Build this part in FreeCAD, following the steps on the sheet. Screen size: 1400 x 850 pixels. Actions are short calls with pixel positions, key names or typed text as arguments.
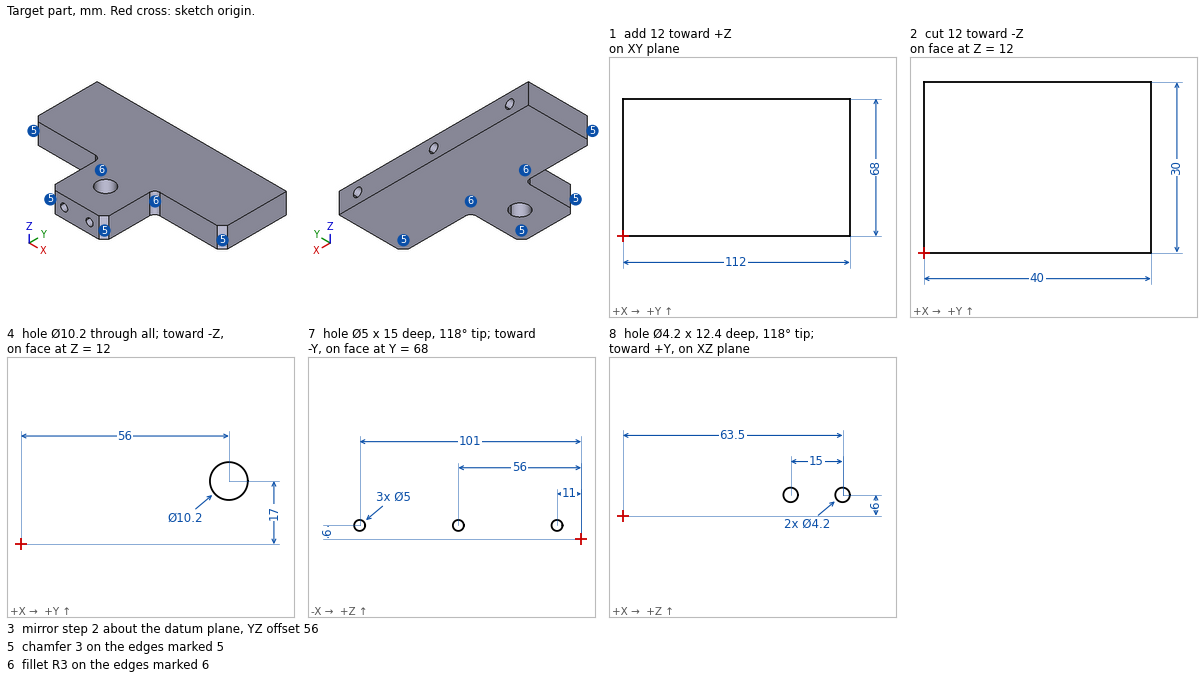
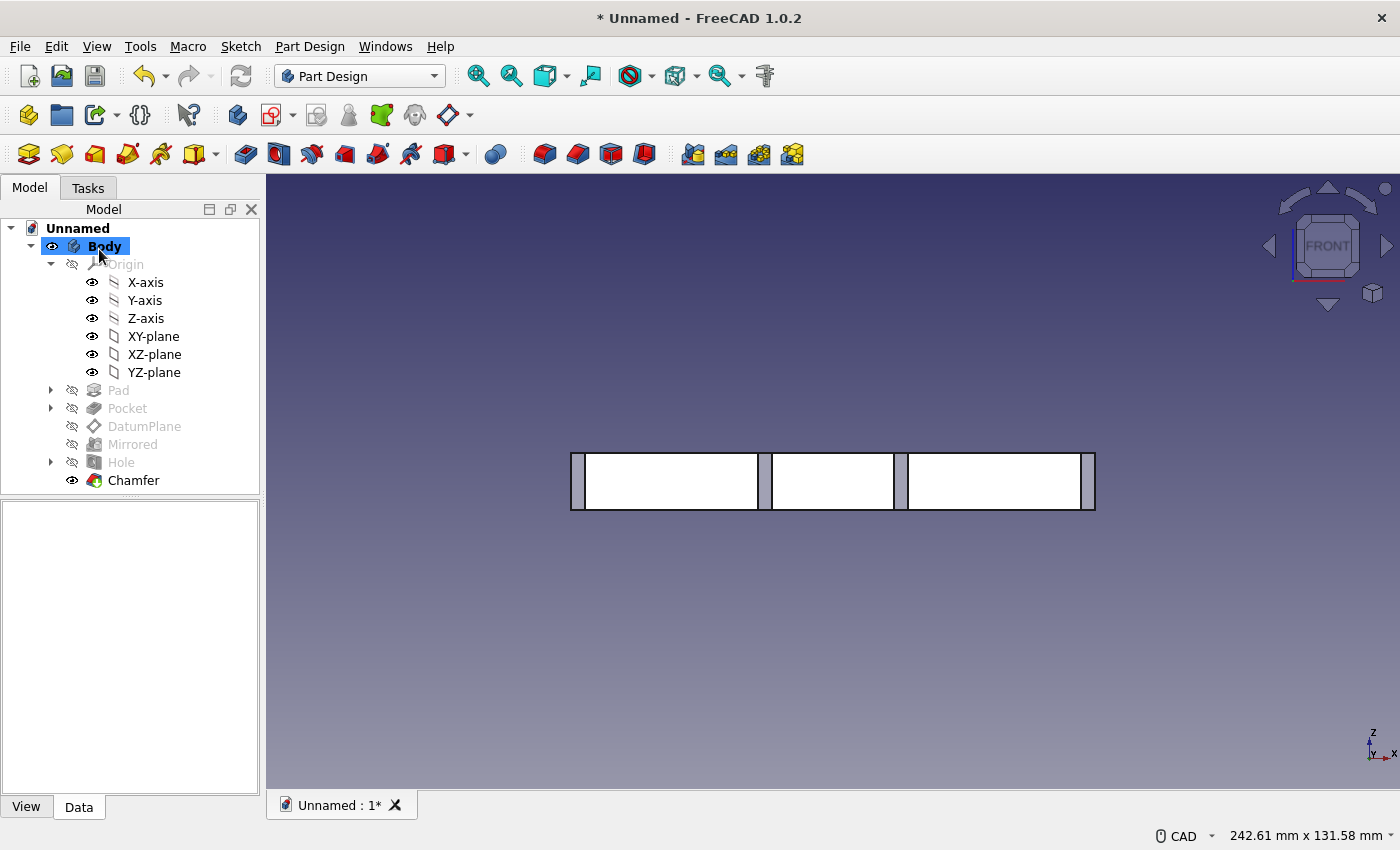
key(3)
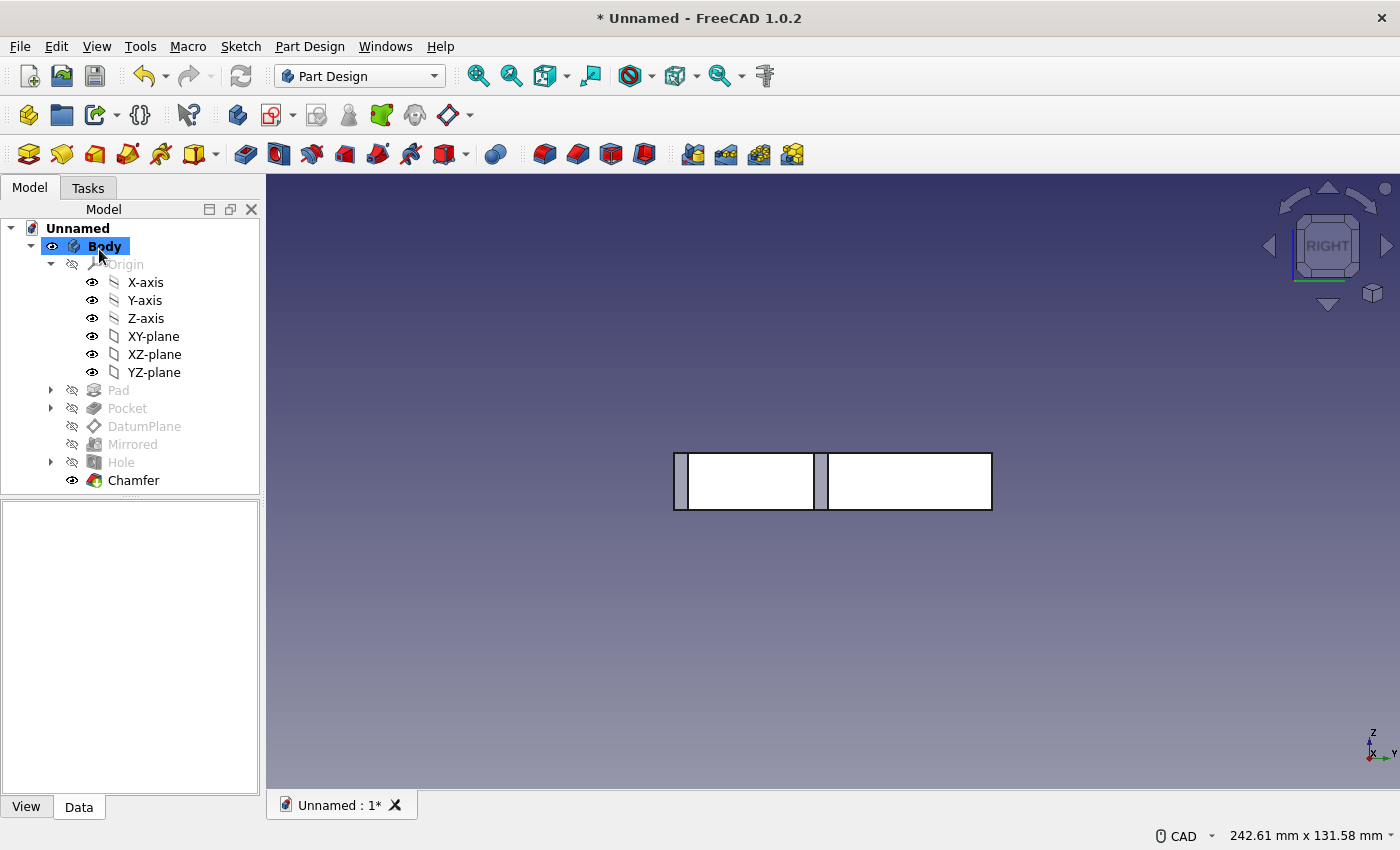
click(479, 76)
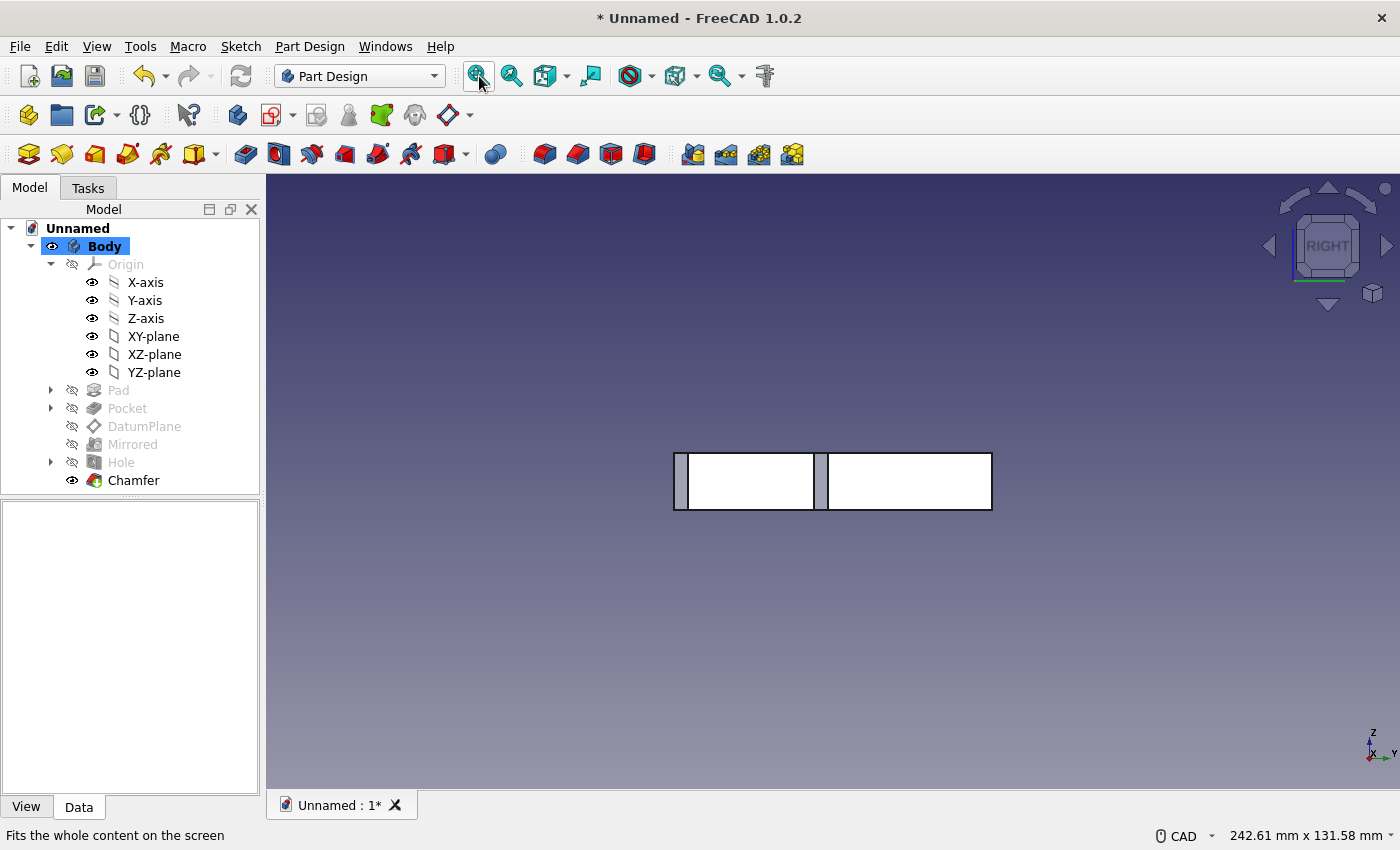
key(5)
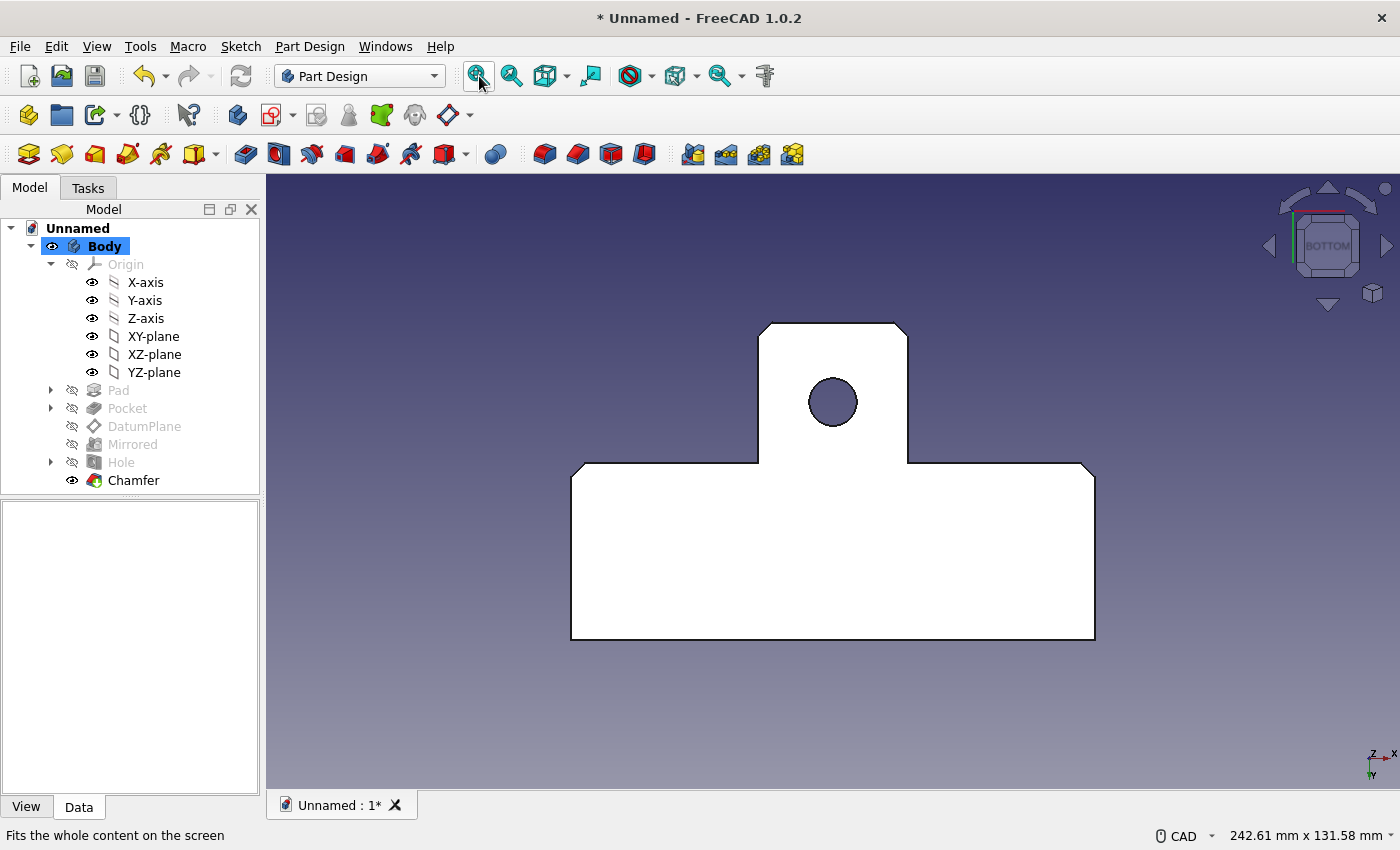
key(4)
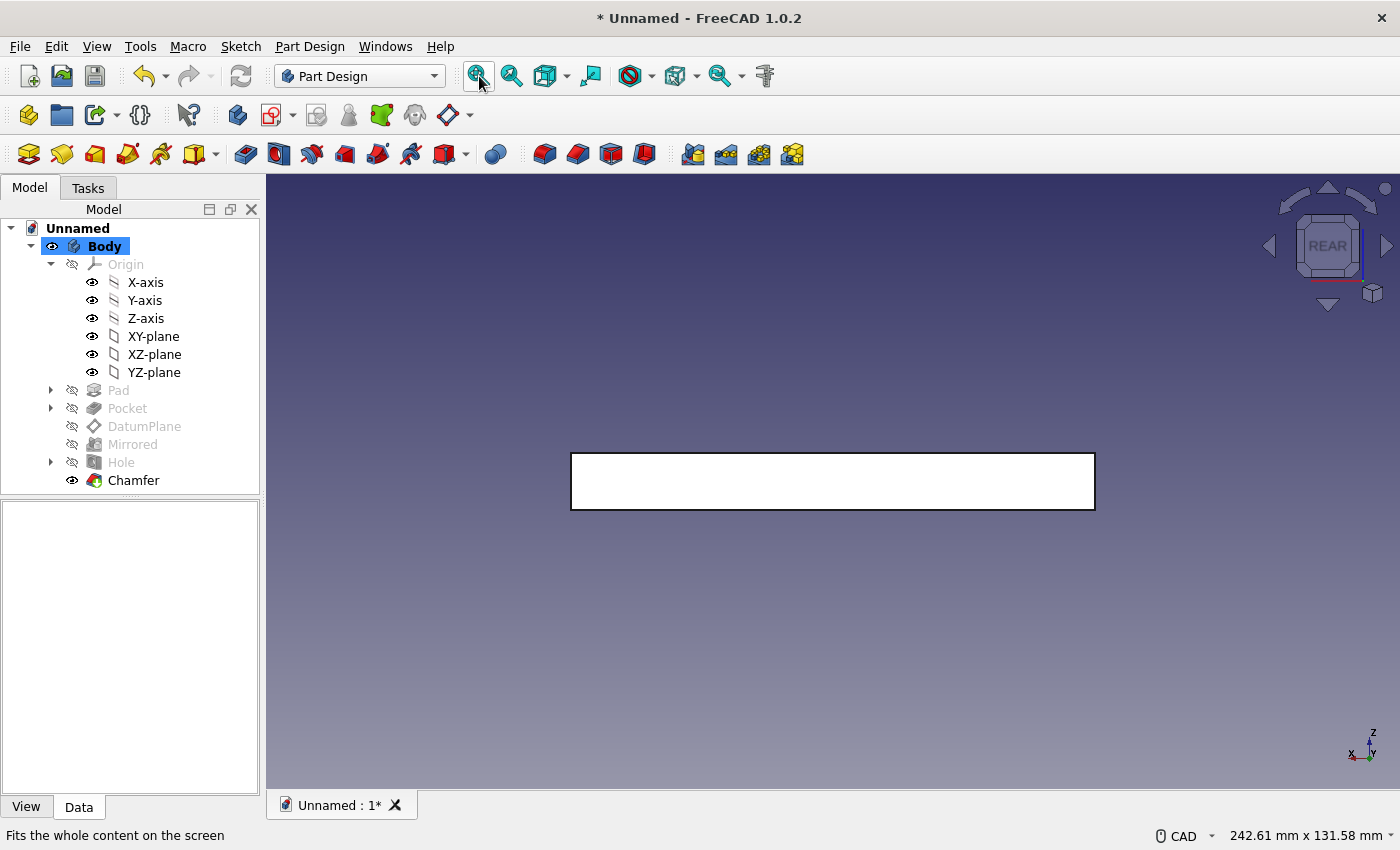
key(6)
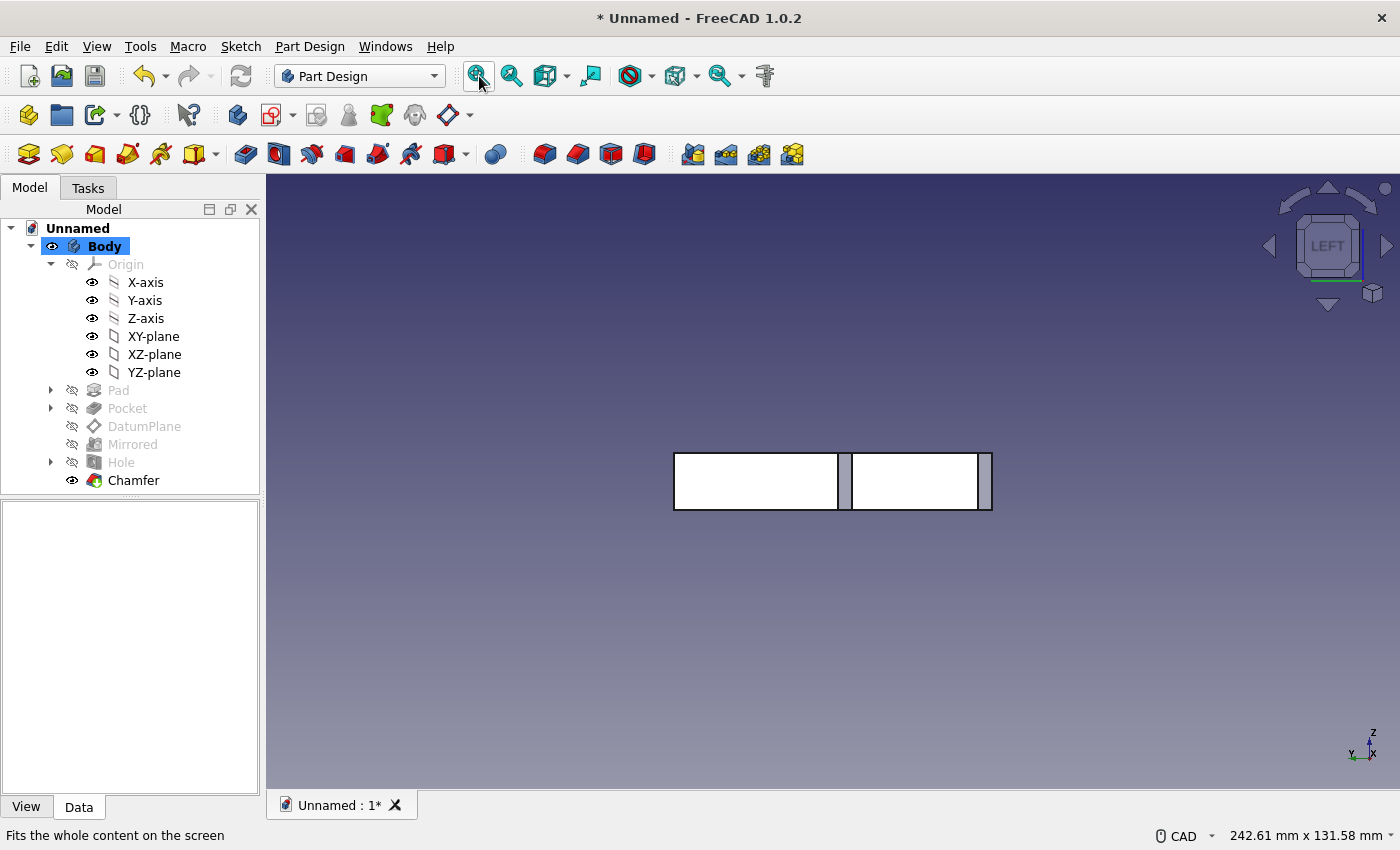
click(479, 76)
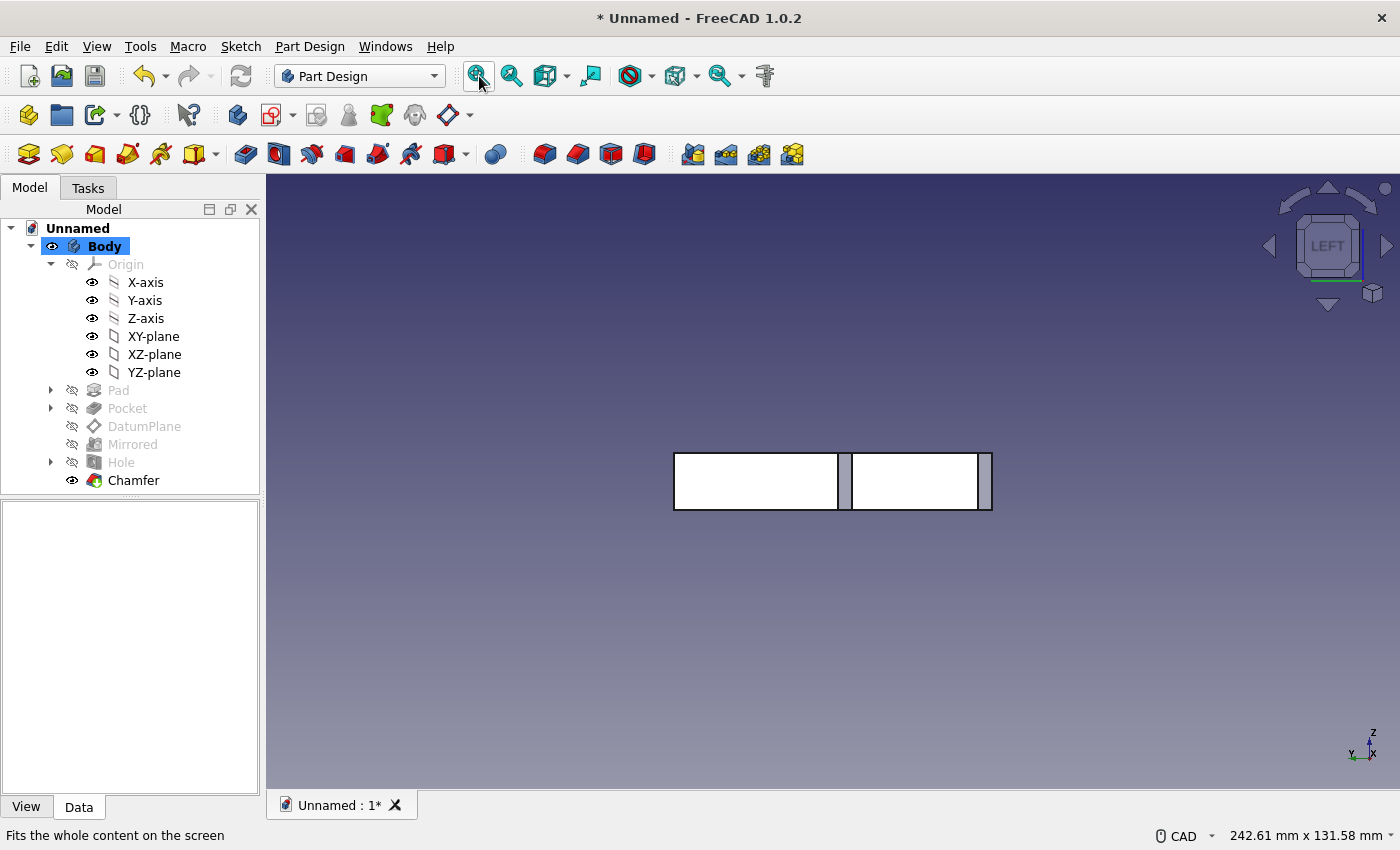
key(v)
key(3)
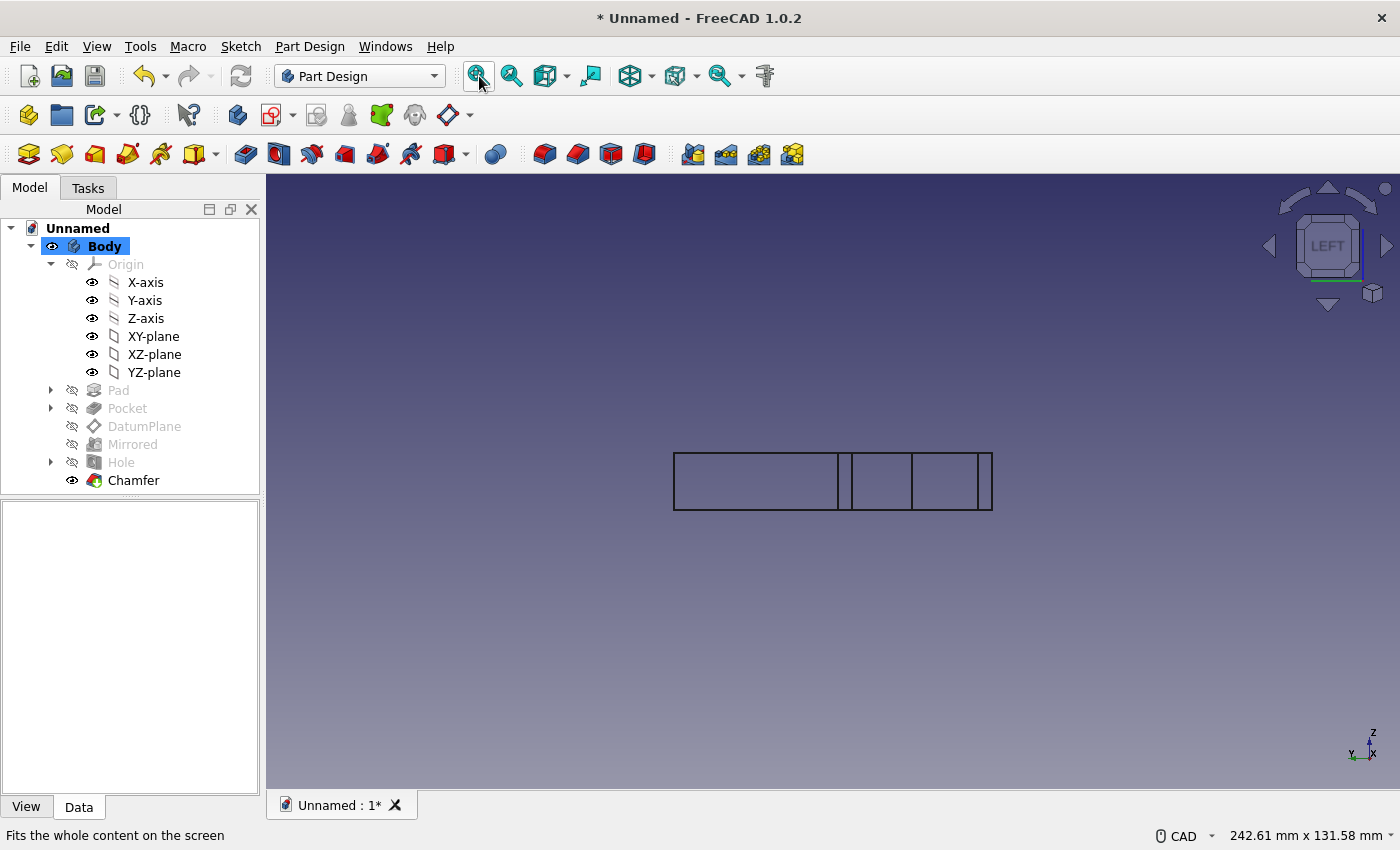
key(0)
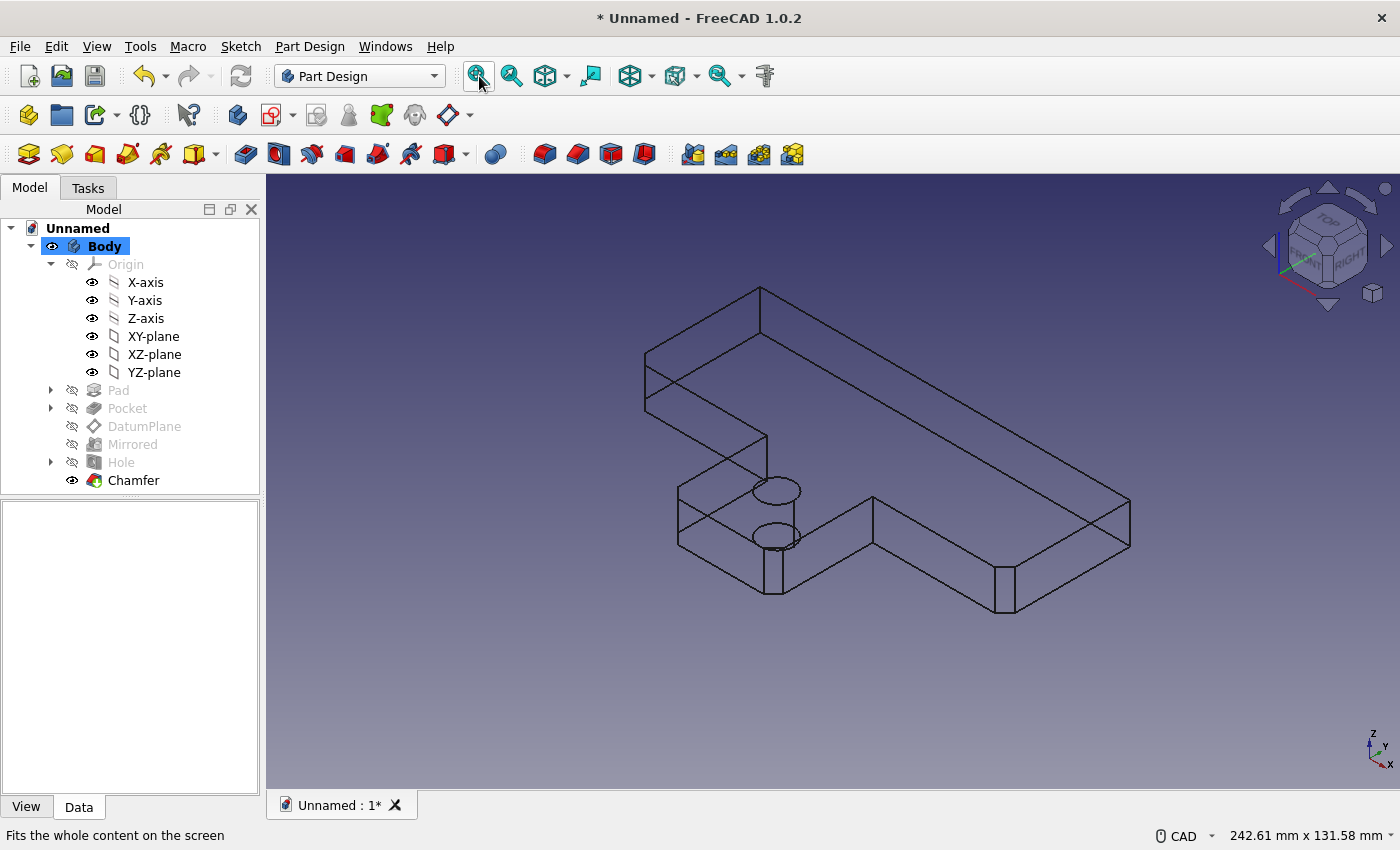
click(767, 458)